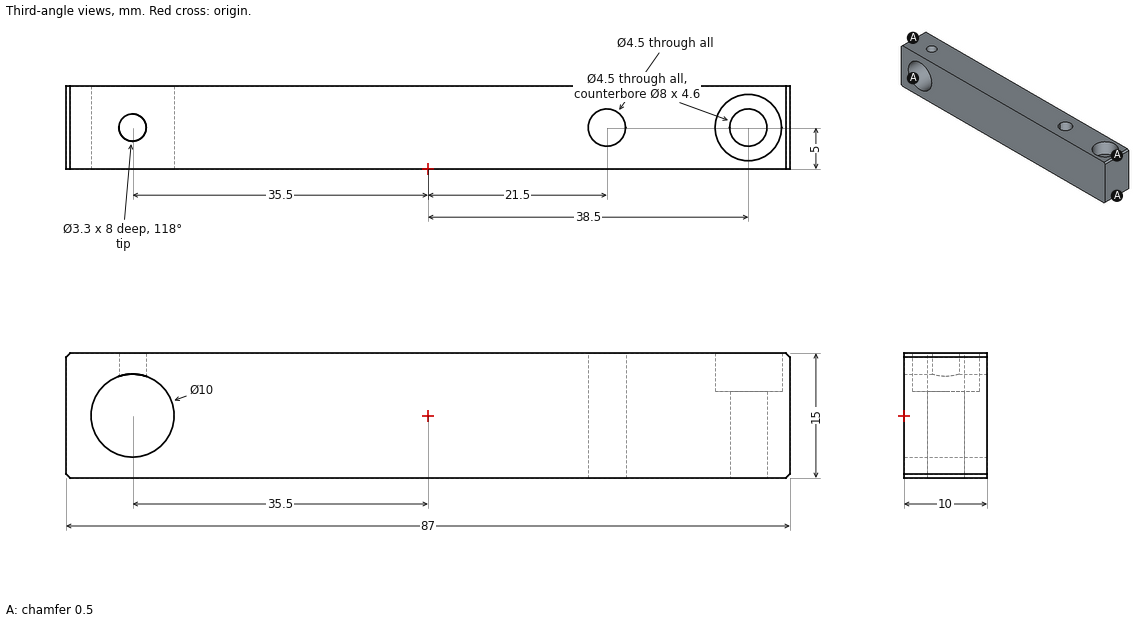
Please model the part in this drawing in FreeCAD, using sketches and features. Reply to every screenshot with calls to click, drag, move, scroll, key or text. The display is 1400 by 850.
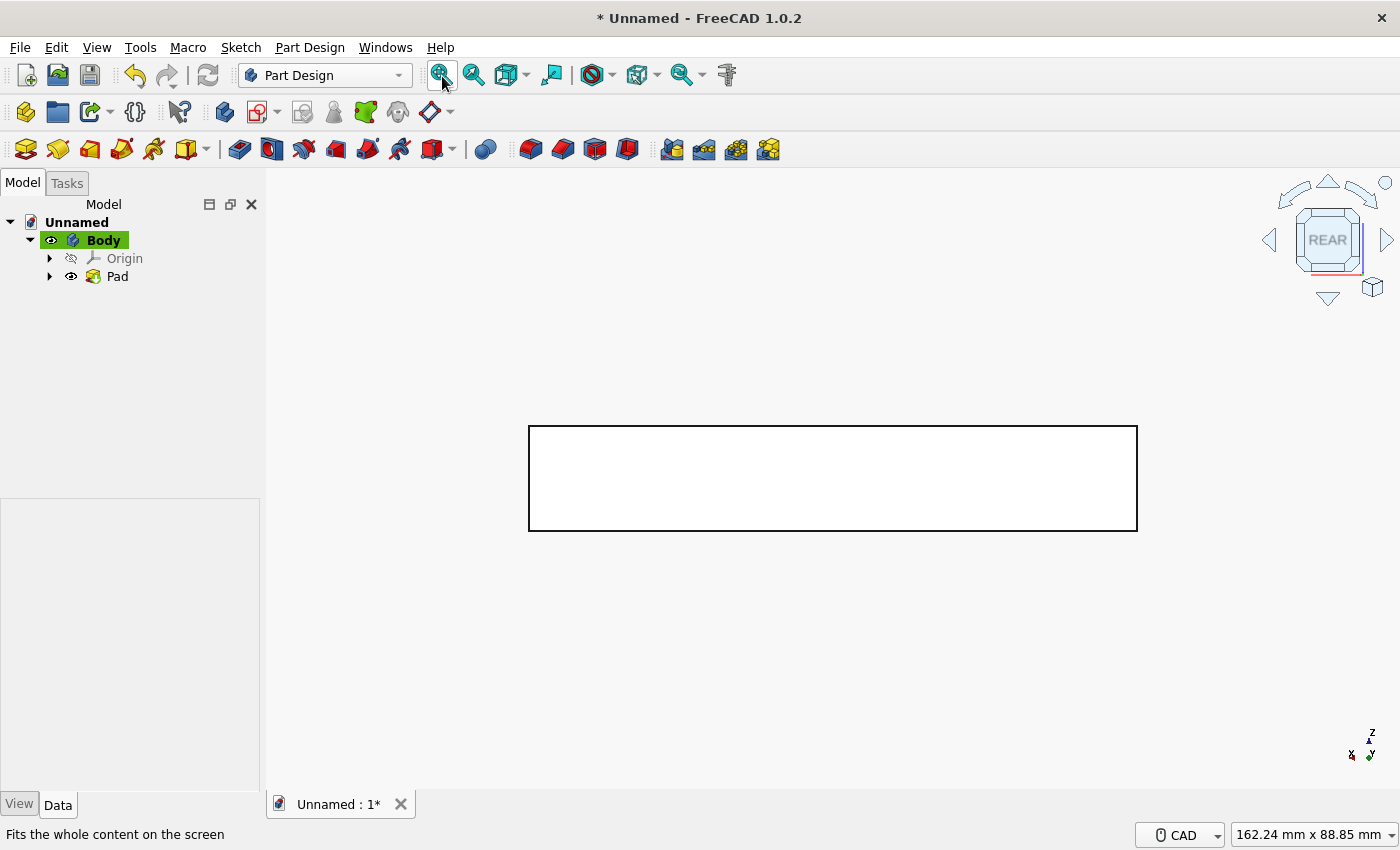
click(659, 478)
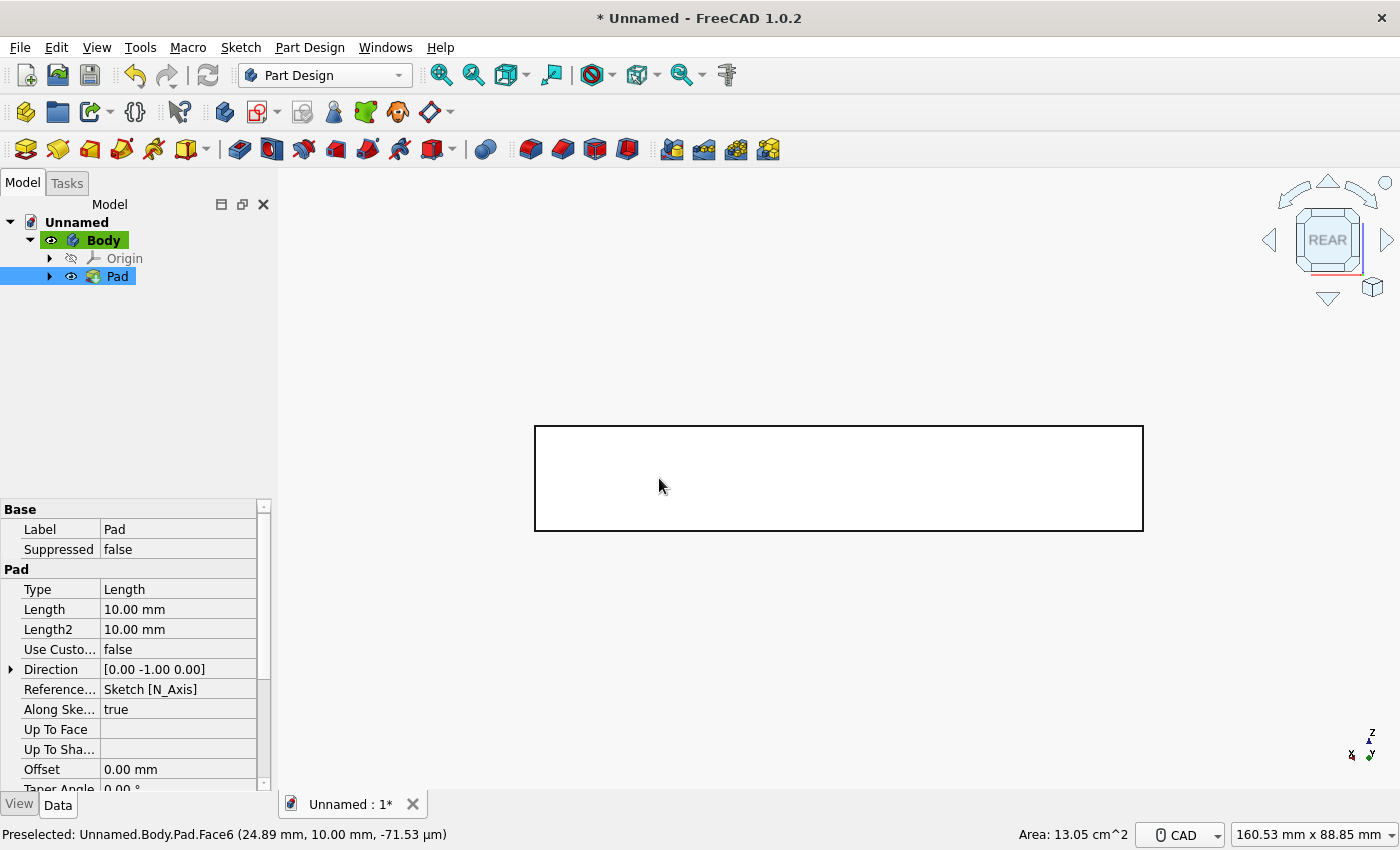
click(258, 112)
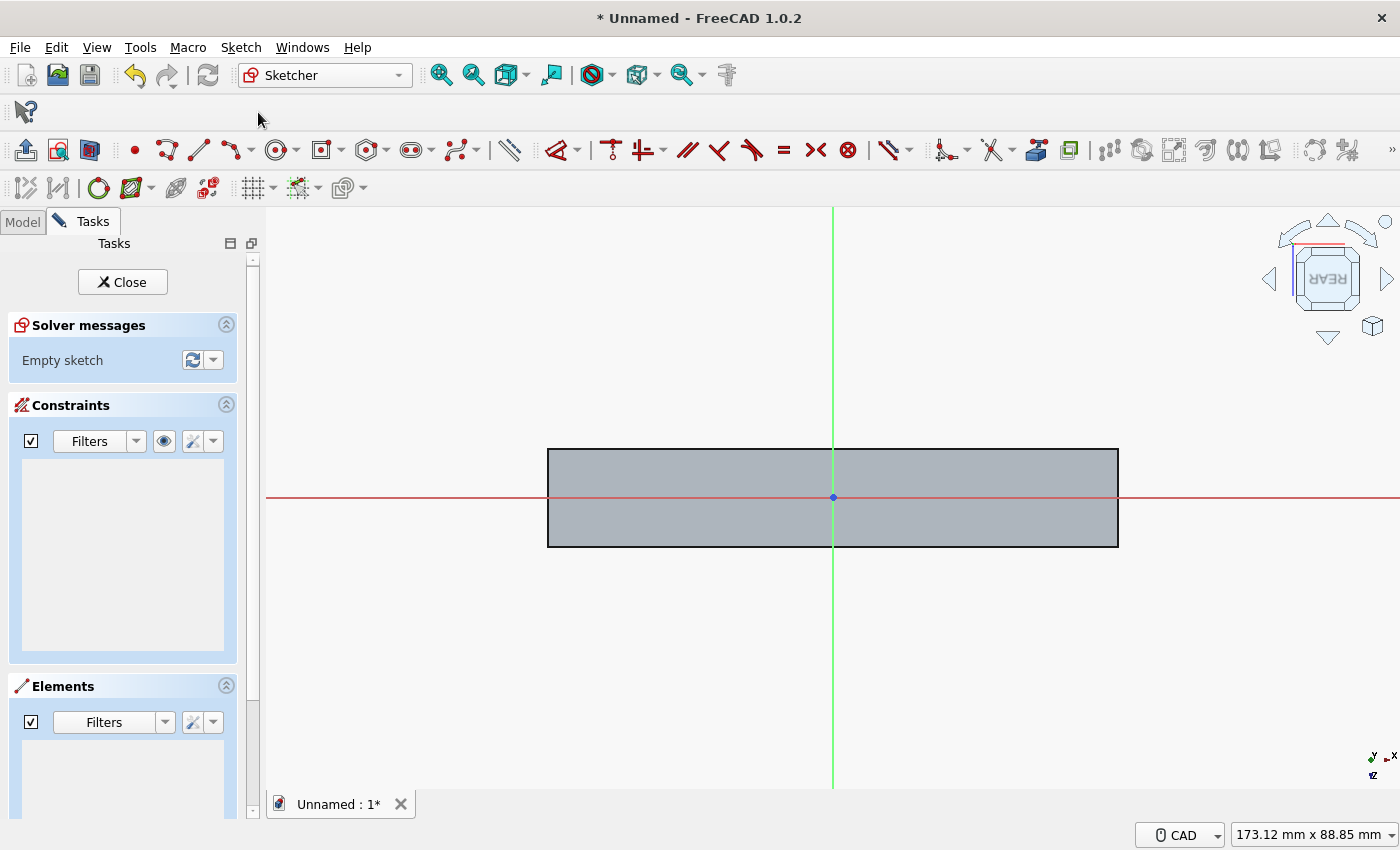
scroll(568, 498, up, 9)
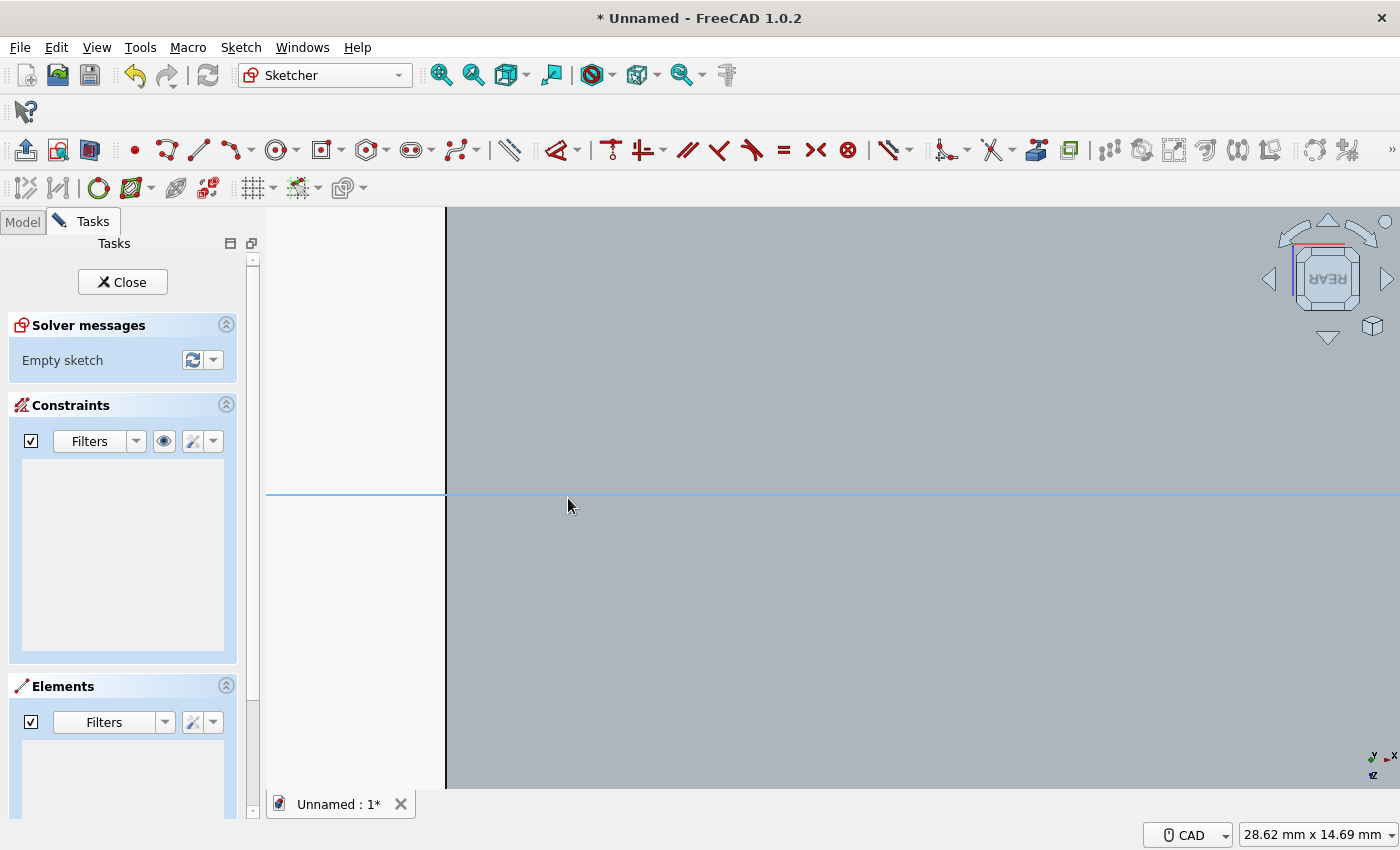
click(276, 150)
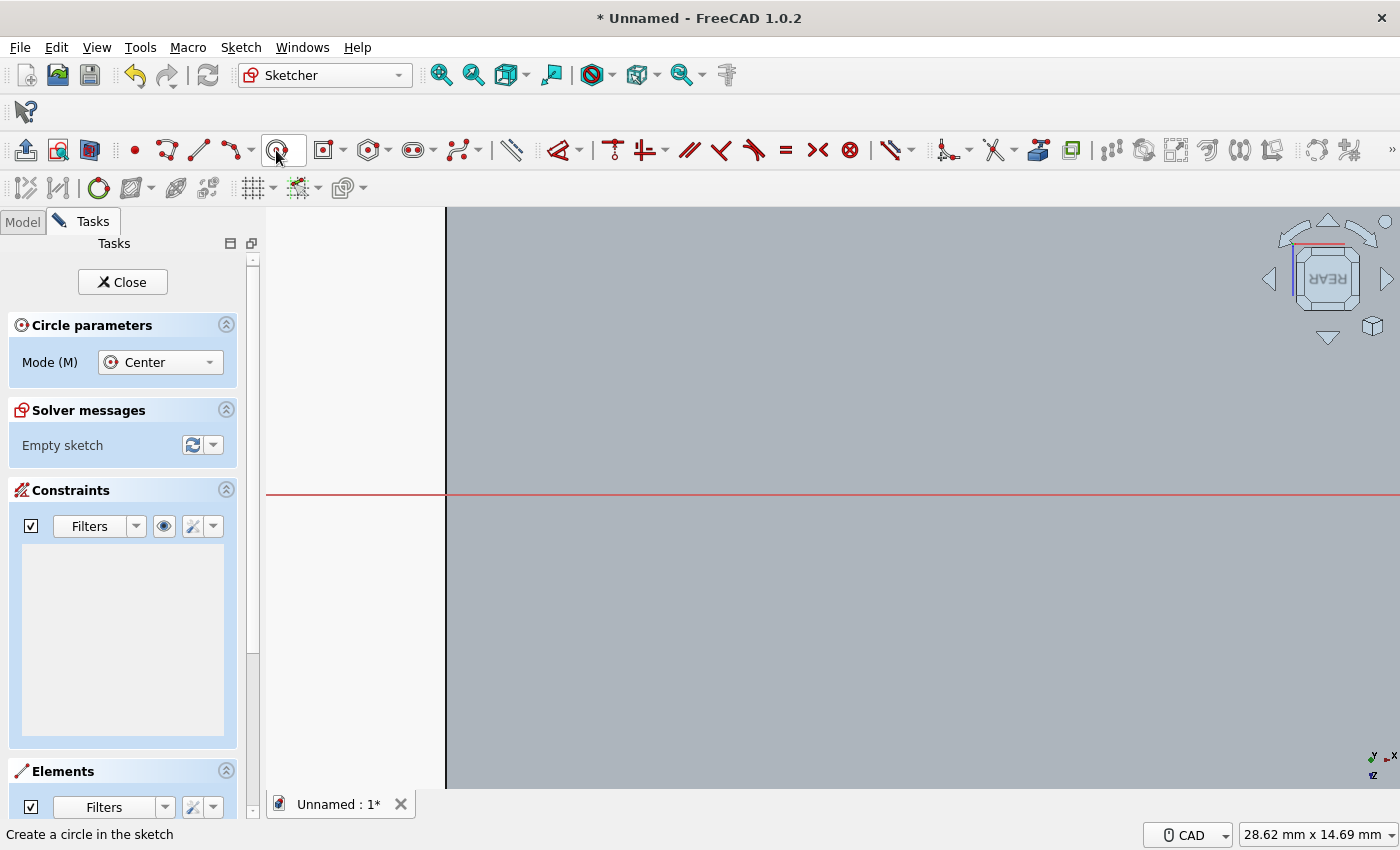
click(763, 495)
click(903, 355)
key(Escape)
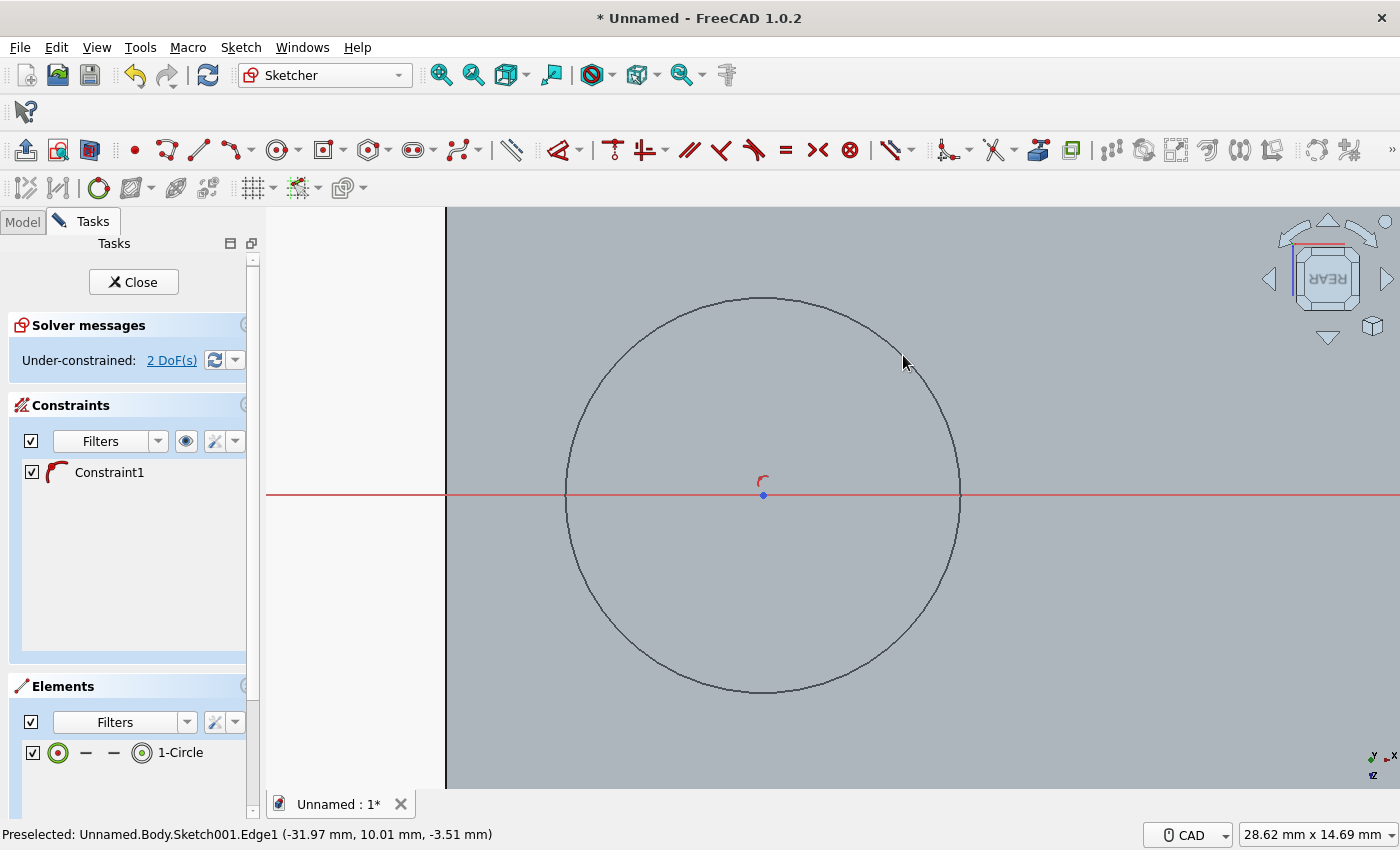
click(558, 150)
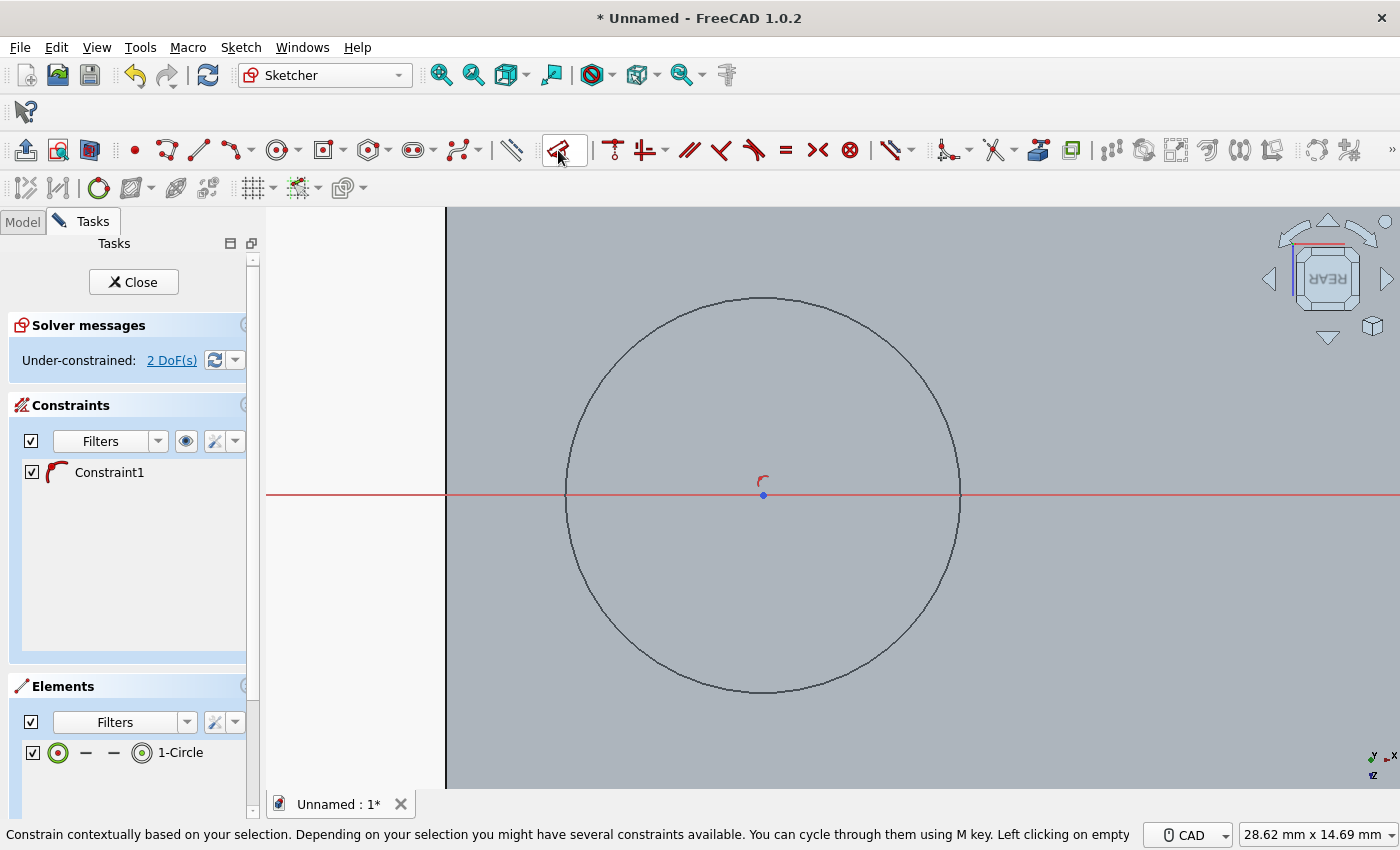
click(902, 355)
click(925, 332)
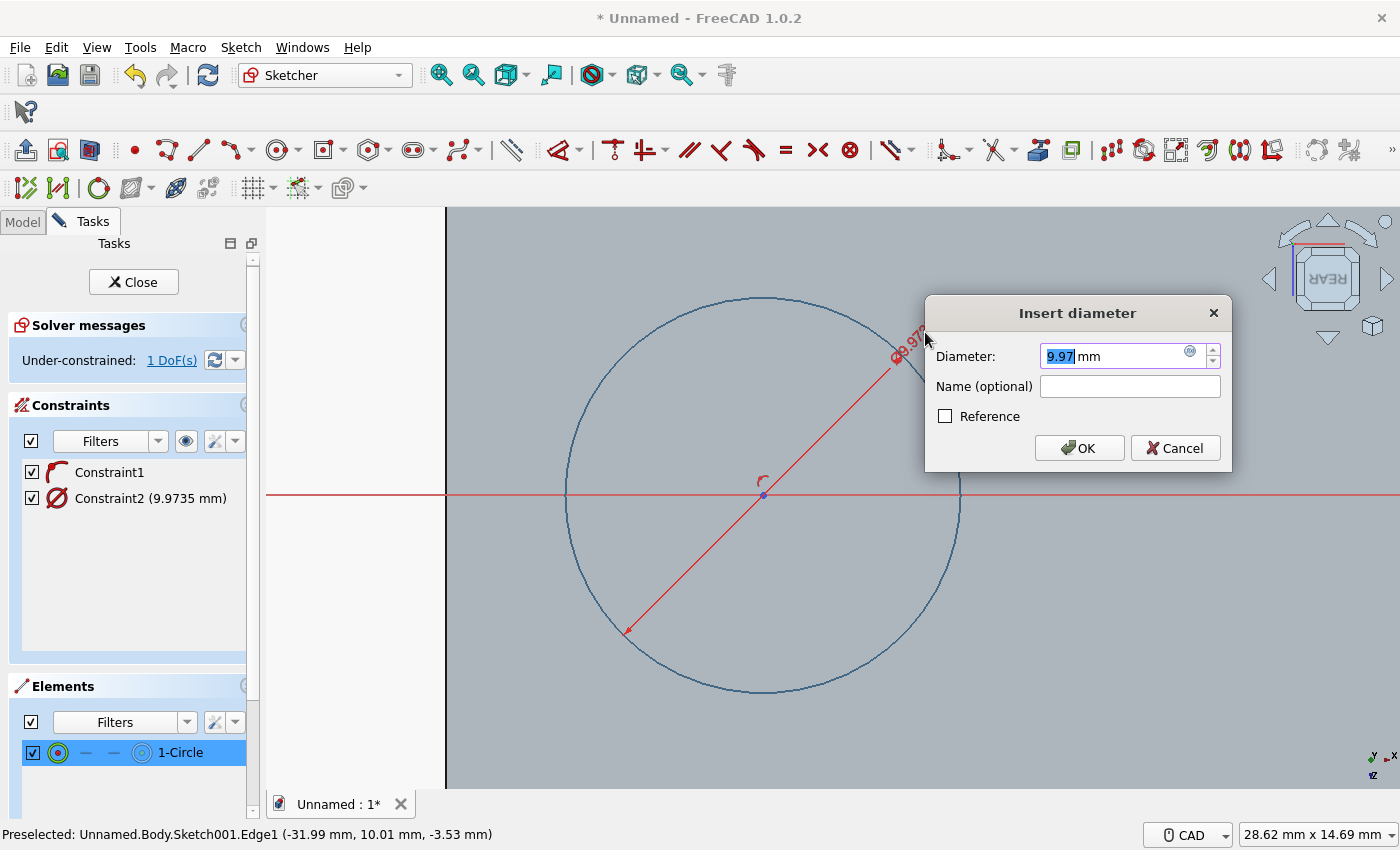
text(10)
key(Return)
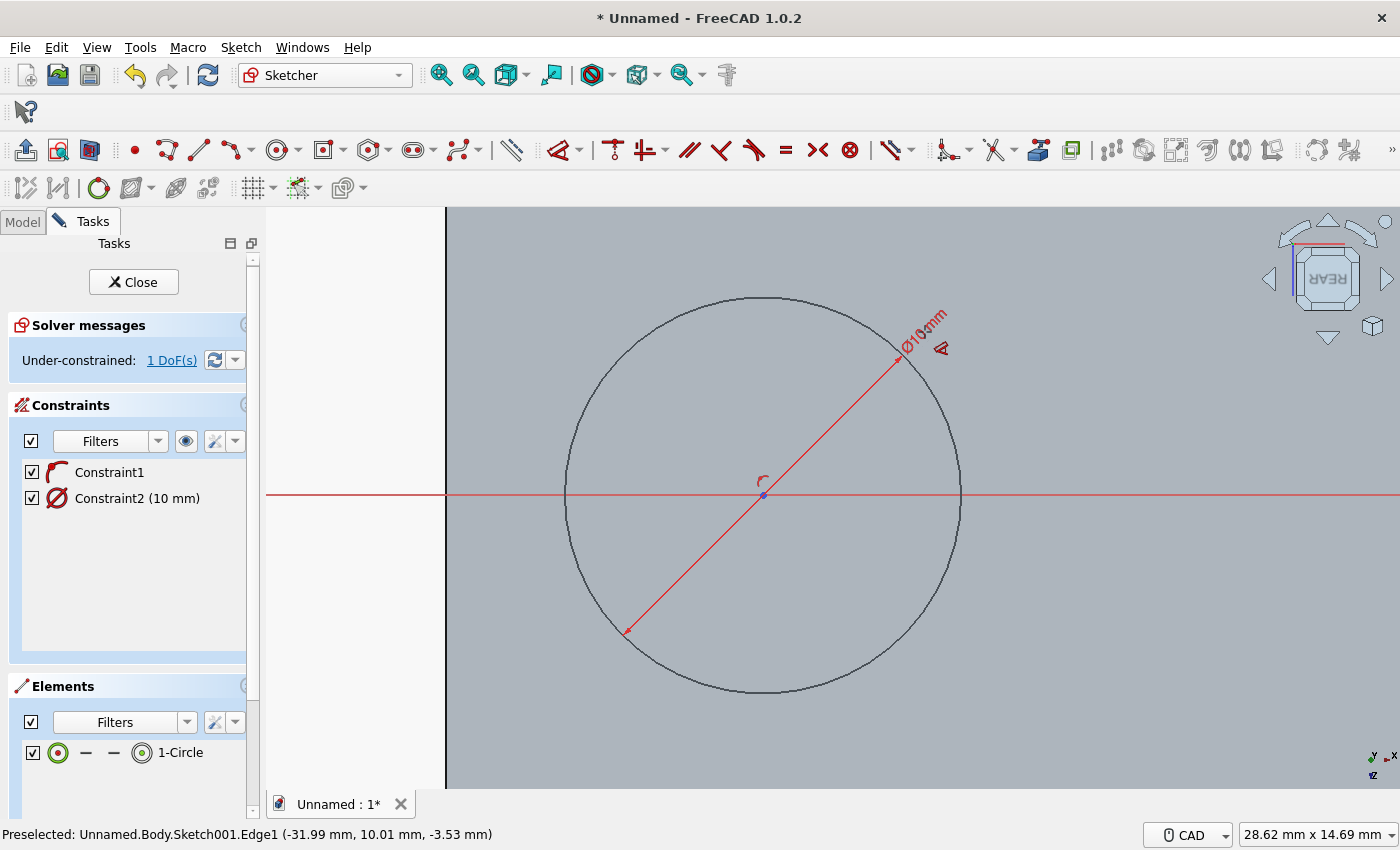
click(763, 495)
click(999, 529)